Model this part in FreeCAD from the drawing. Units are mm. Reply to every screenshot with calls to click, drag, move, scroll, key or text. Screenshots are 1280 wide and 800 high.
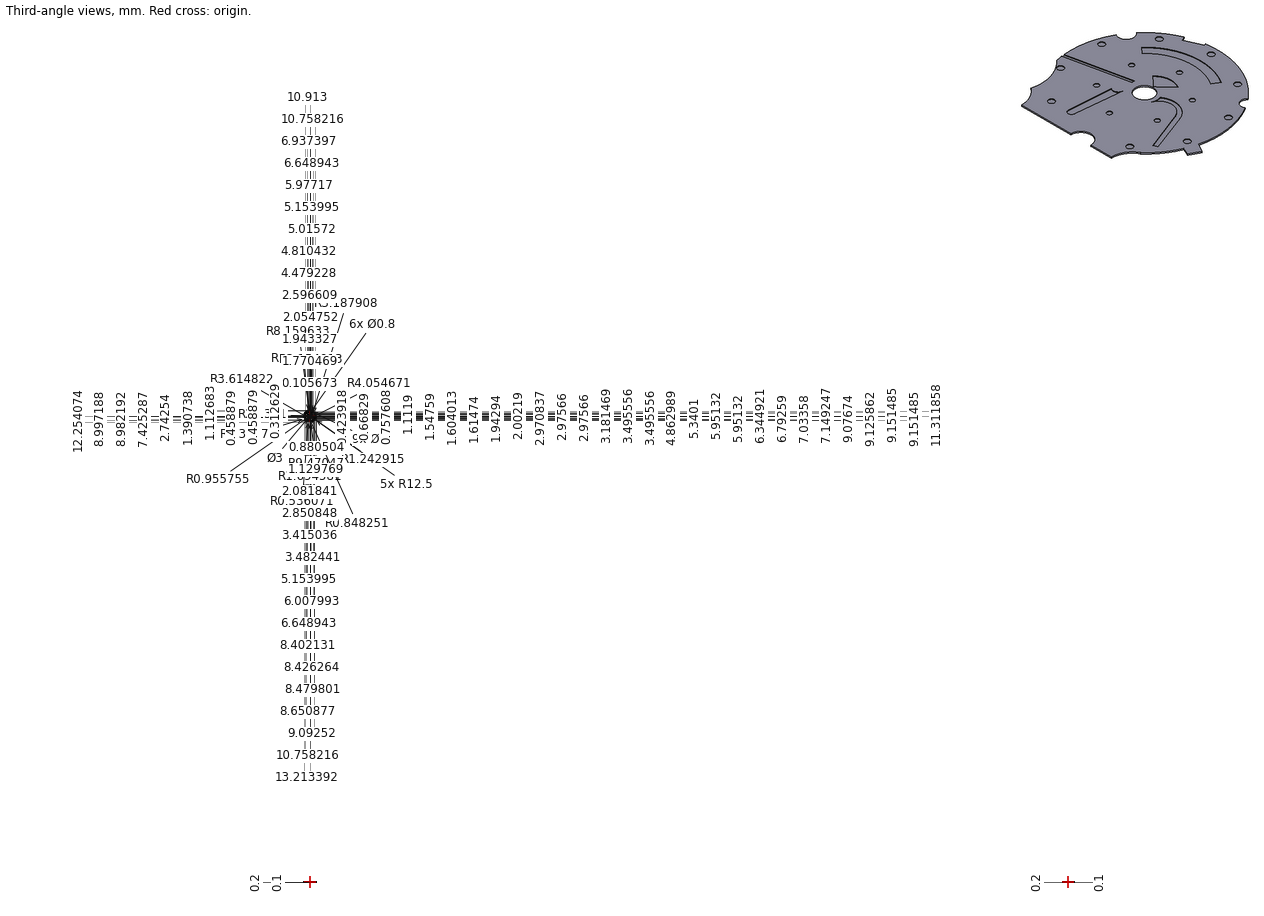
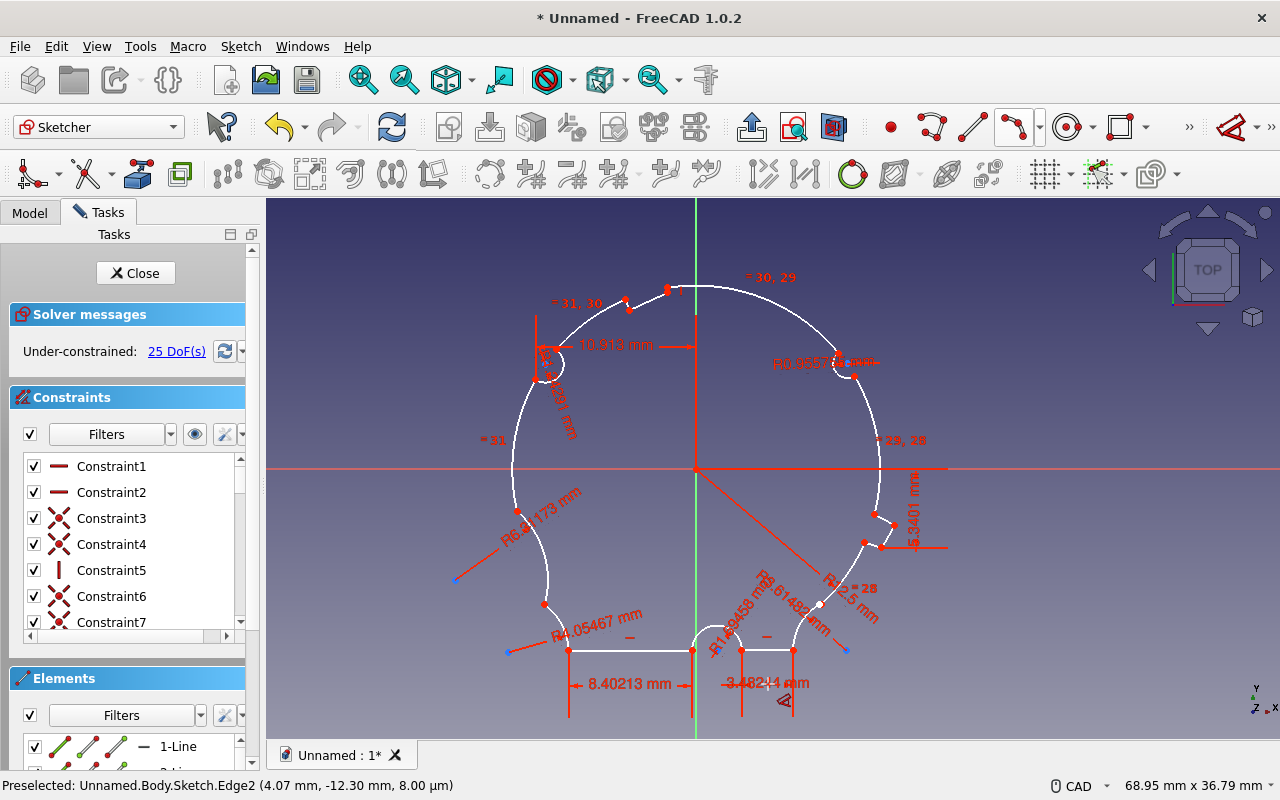
scroll(668, 290, up, 11)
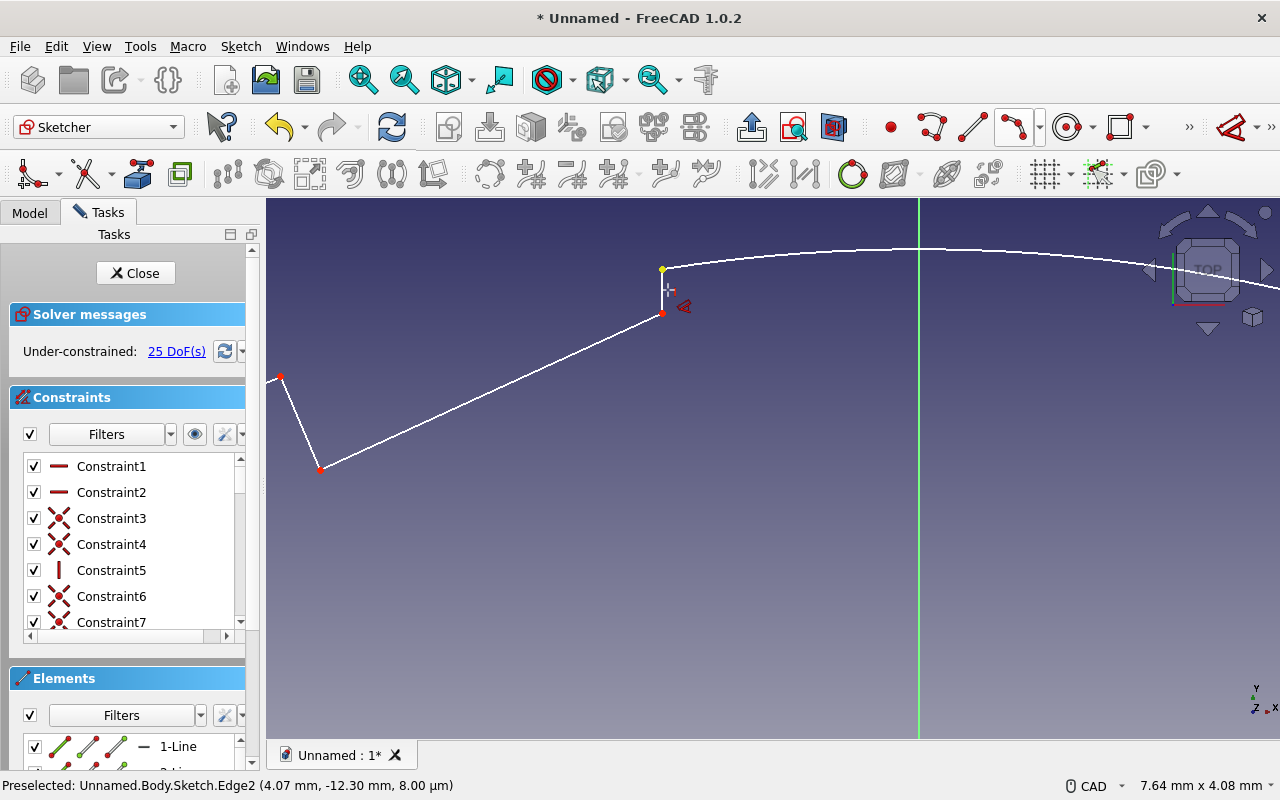
click(662, 291)
click(628, 291)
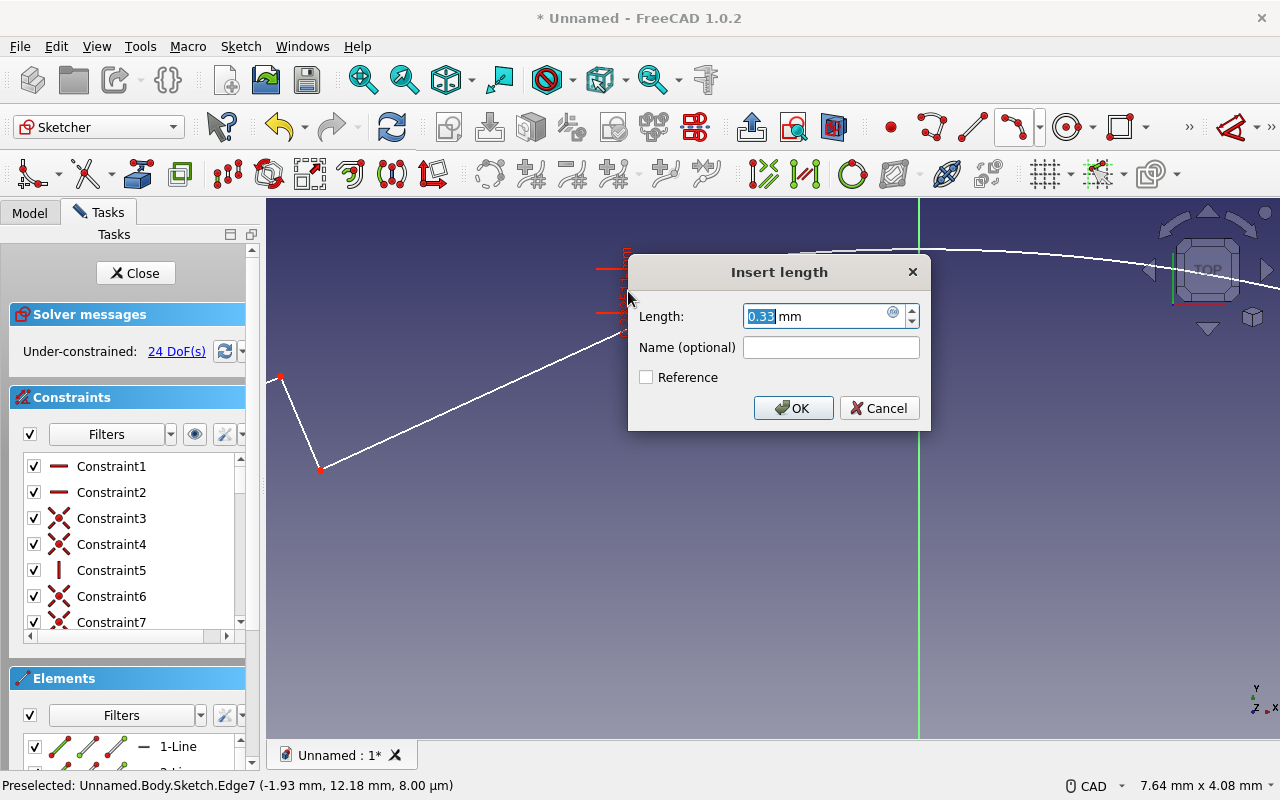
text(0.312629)
key(Return)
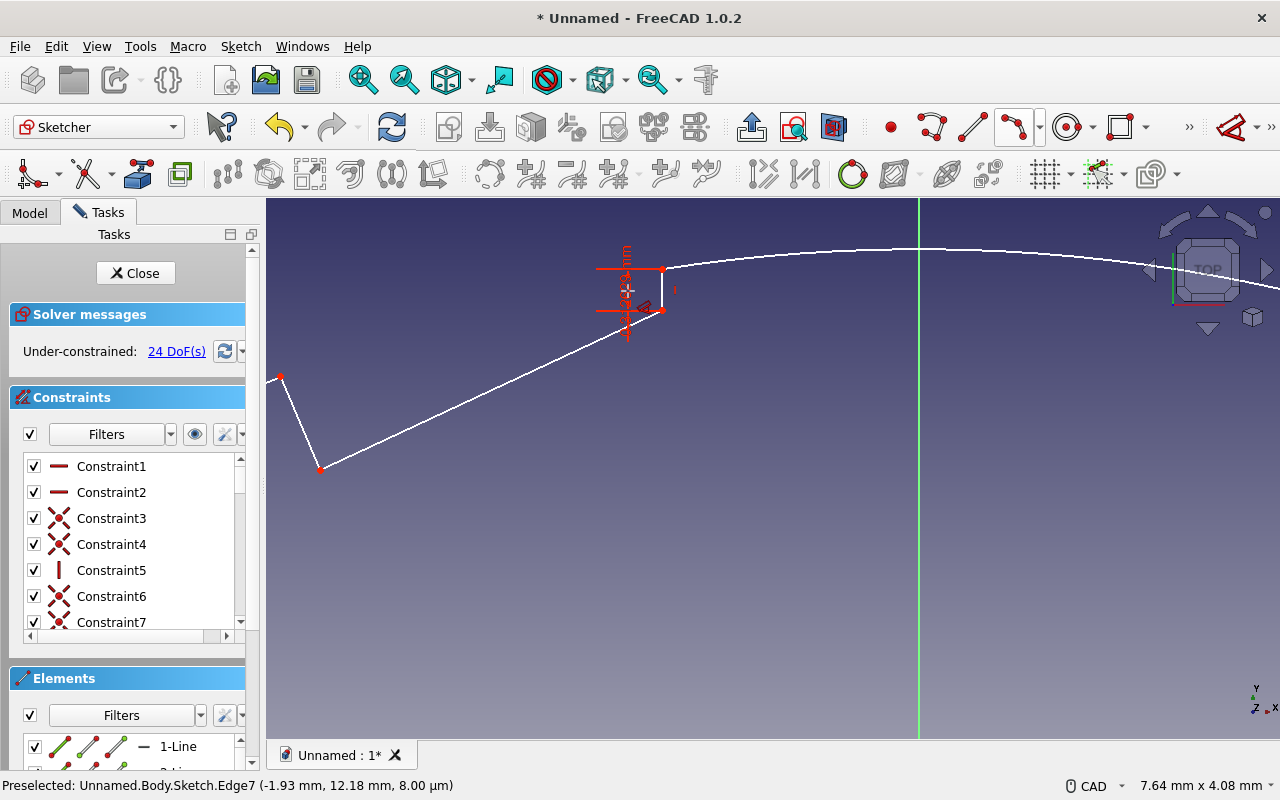
scroll(668, 290, down, 11)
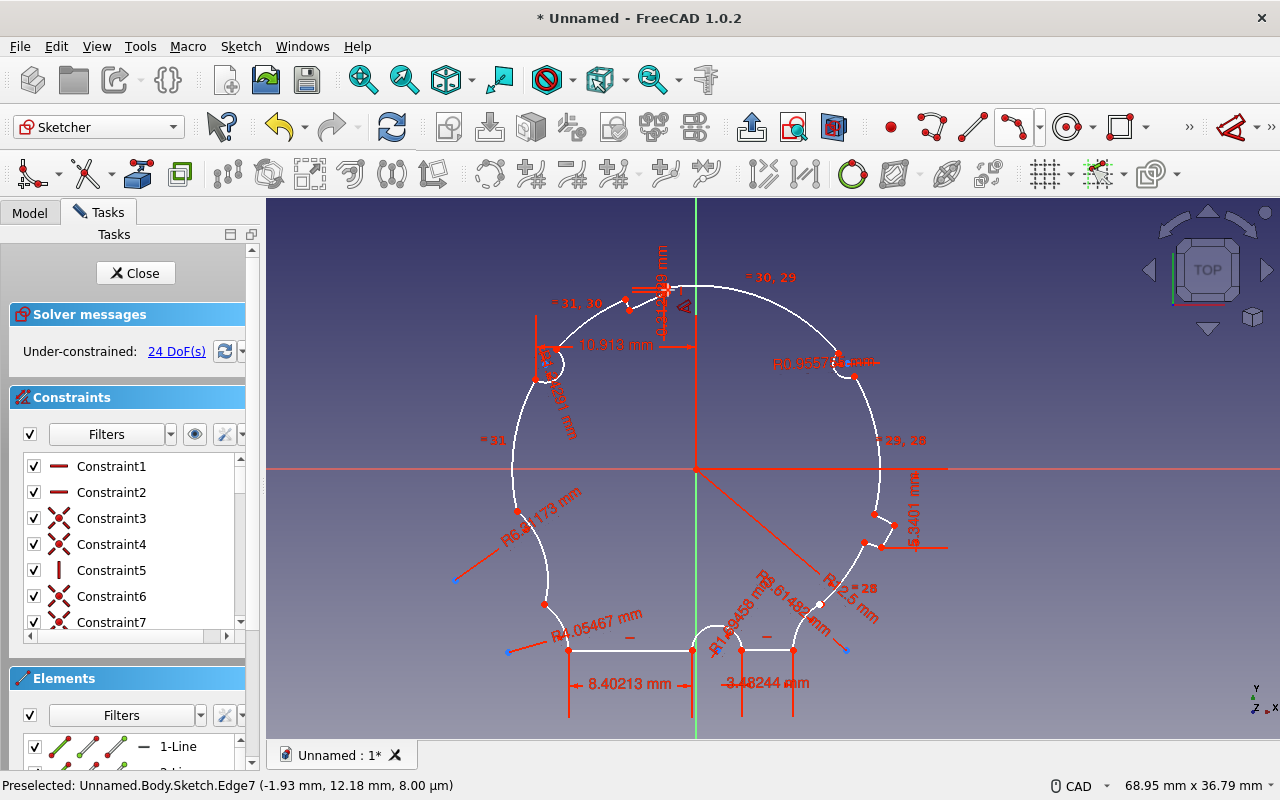
click(517, 511)
click(483, 490)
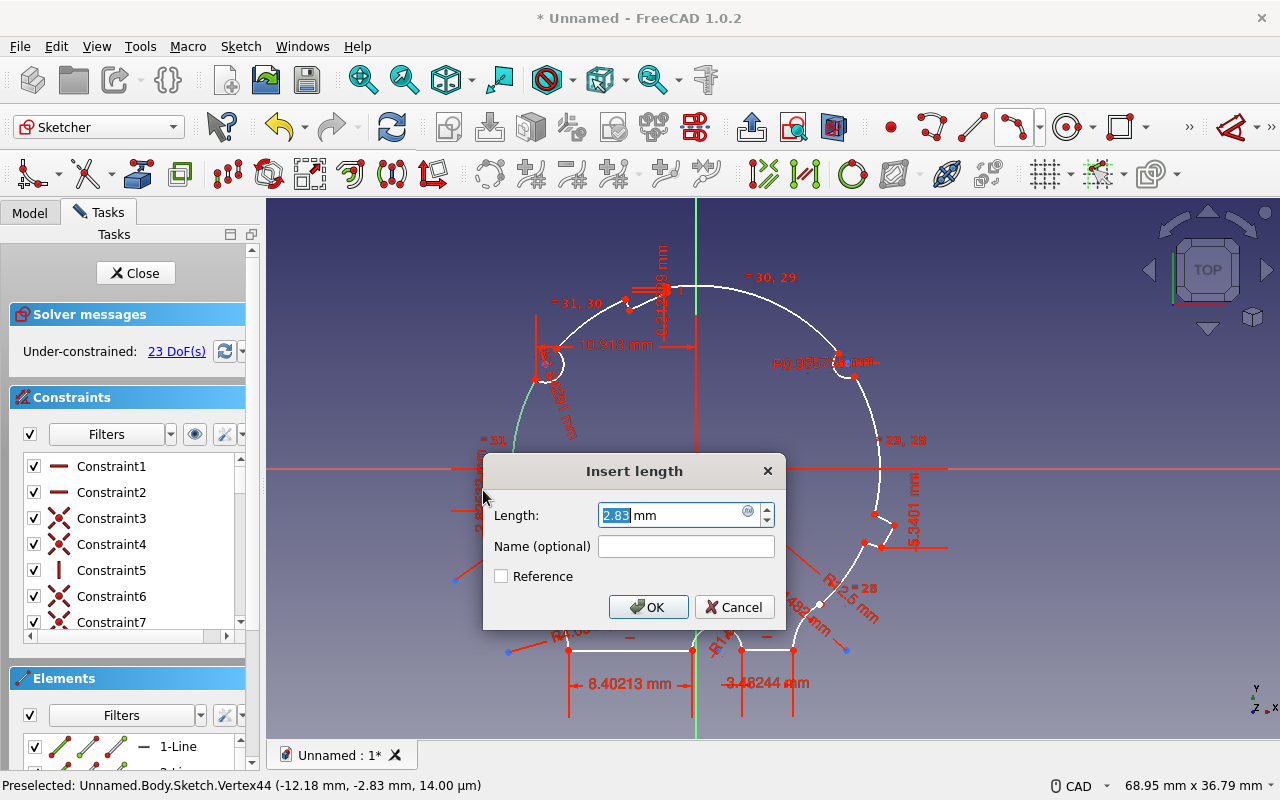
text(2.74254)
key(Return)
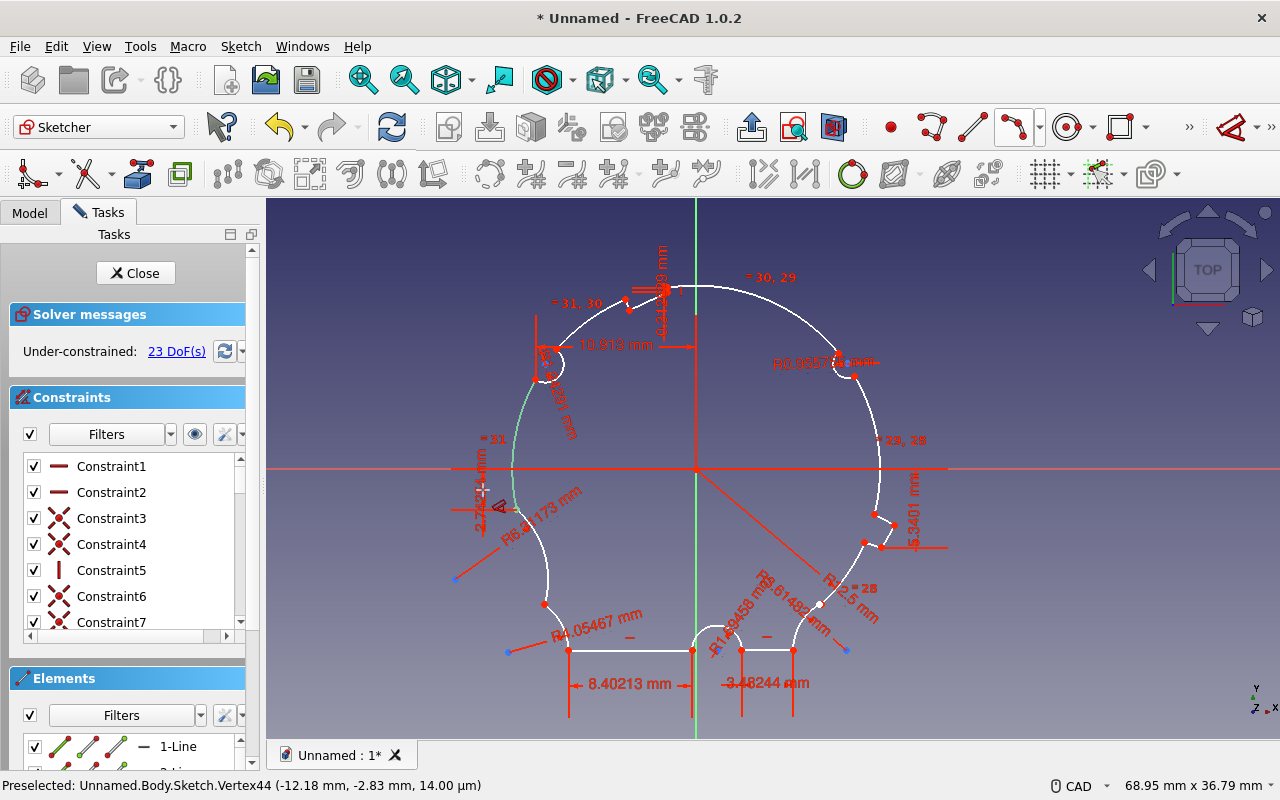
scroll(887, 539, up, 3)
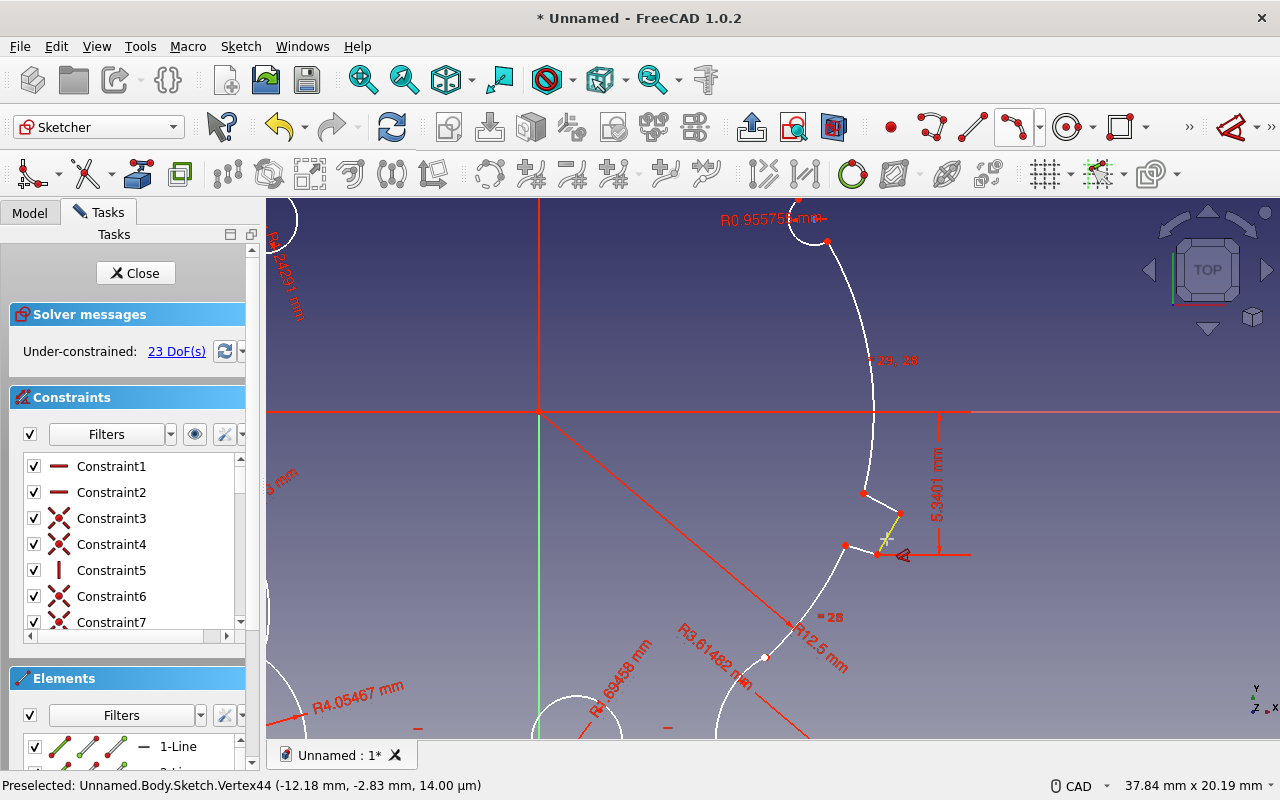
click(887, 538)
click(935, 534)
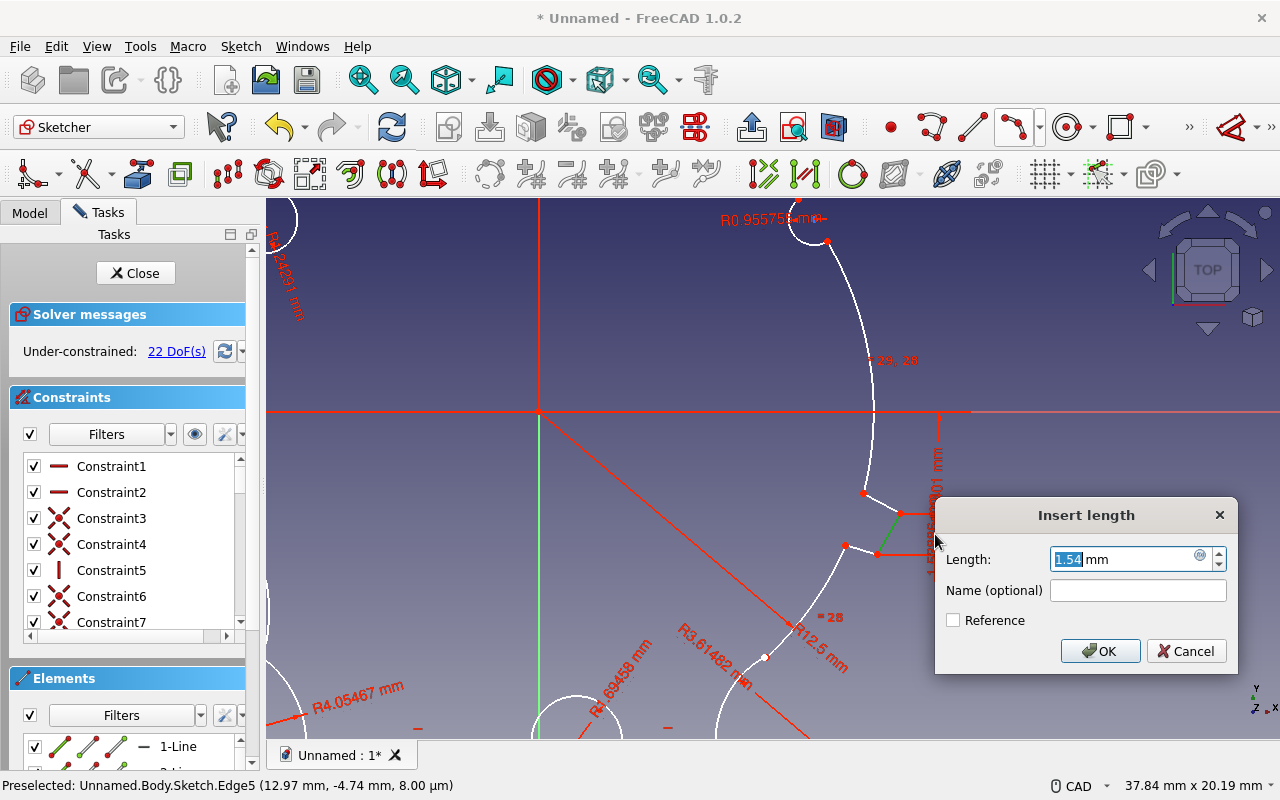
text(1.61474)
key(Return)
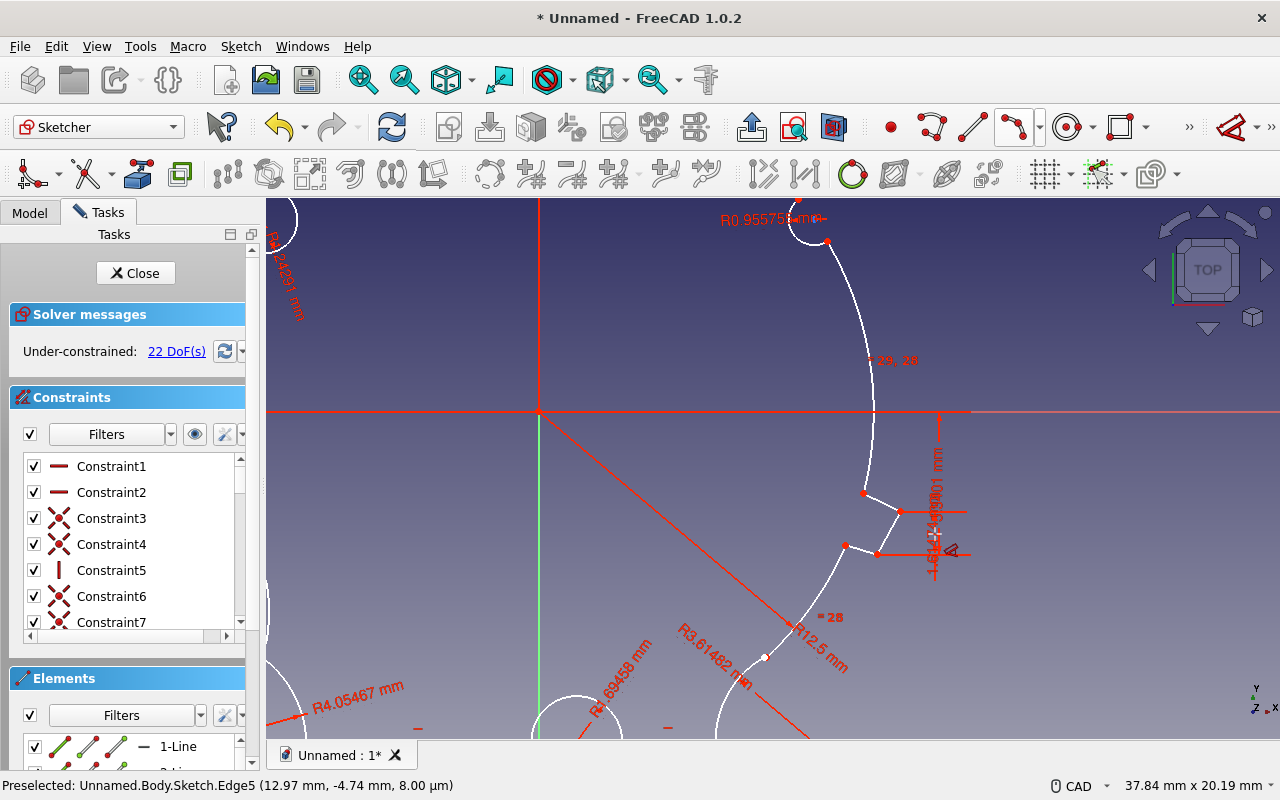
scroll(887, 539, down, 3)